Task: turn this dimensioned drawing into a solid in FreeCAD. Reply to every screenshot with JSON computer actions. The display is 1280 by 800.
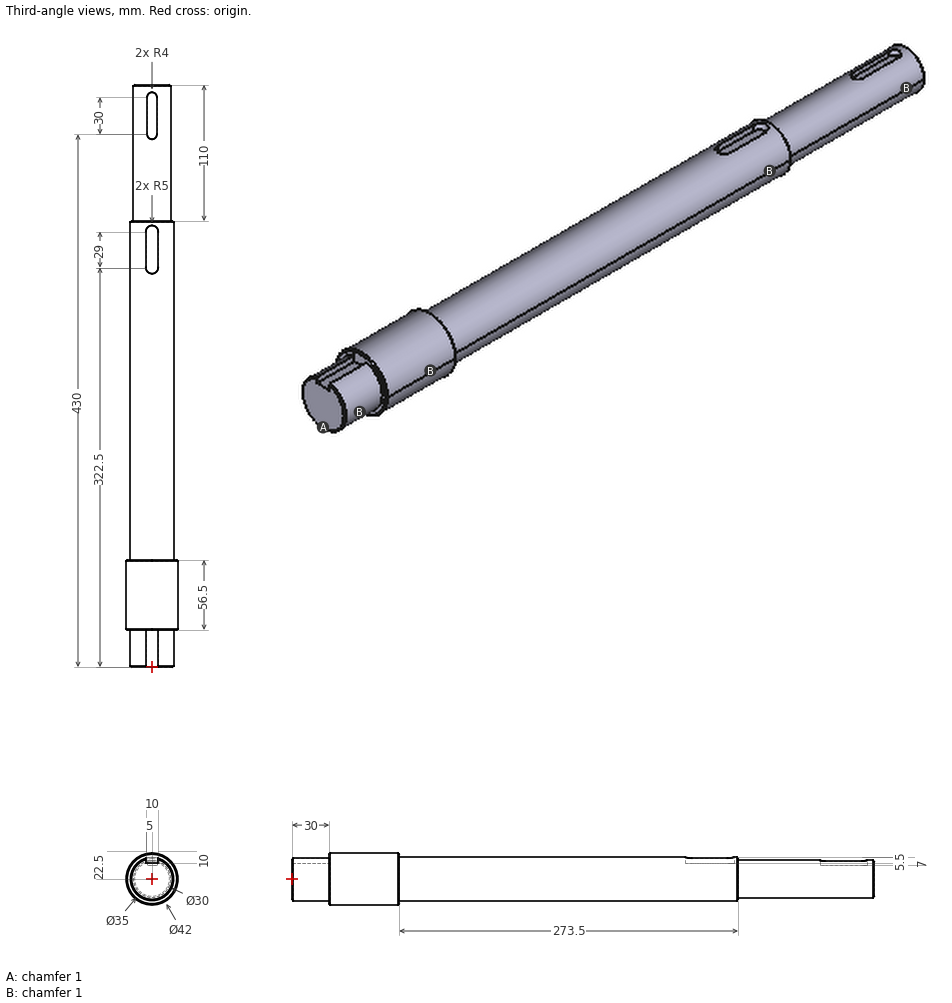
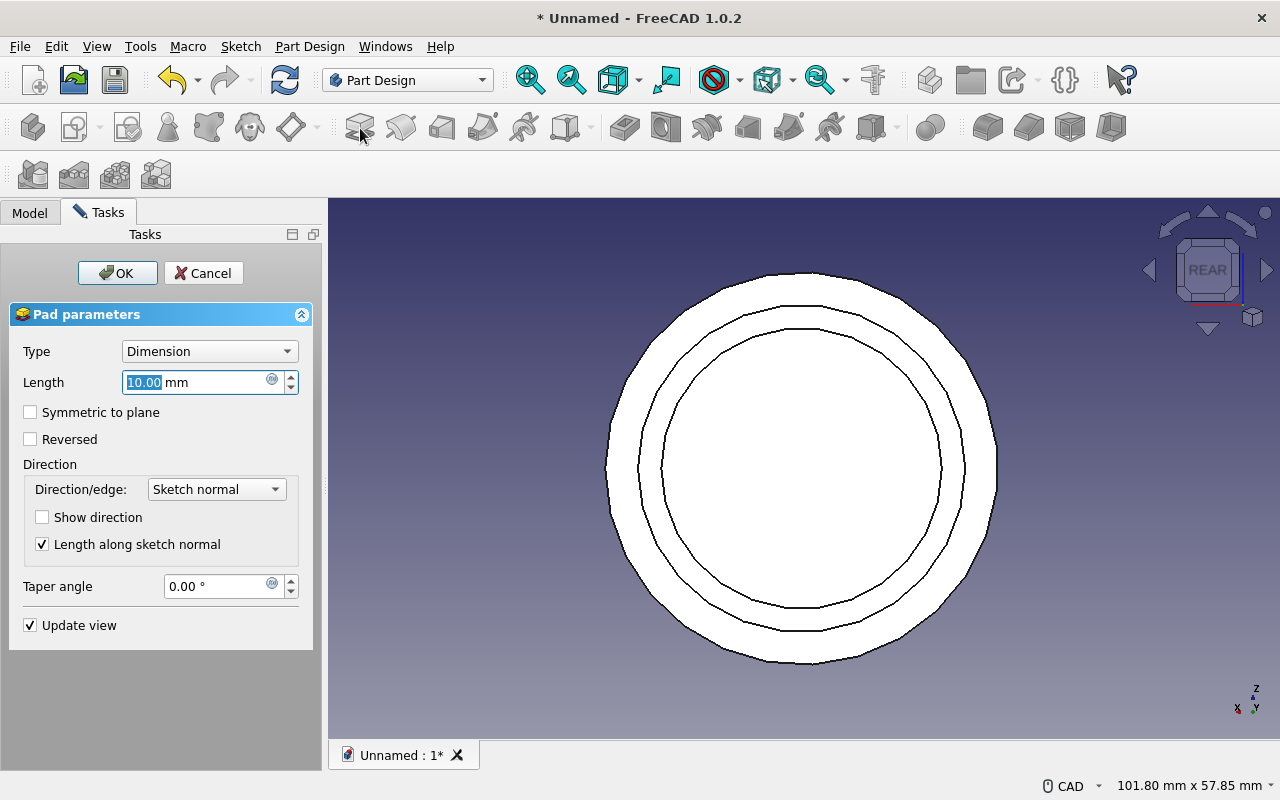
{"action": "type", "text": "110"}
{"action": "key", "text": "Tab"}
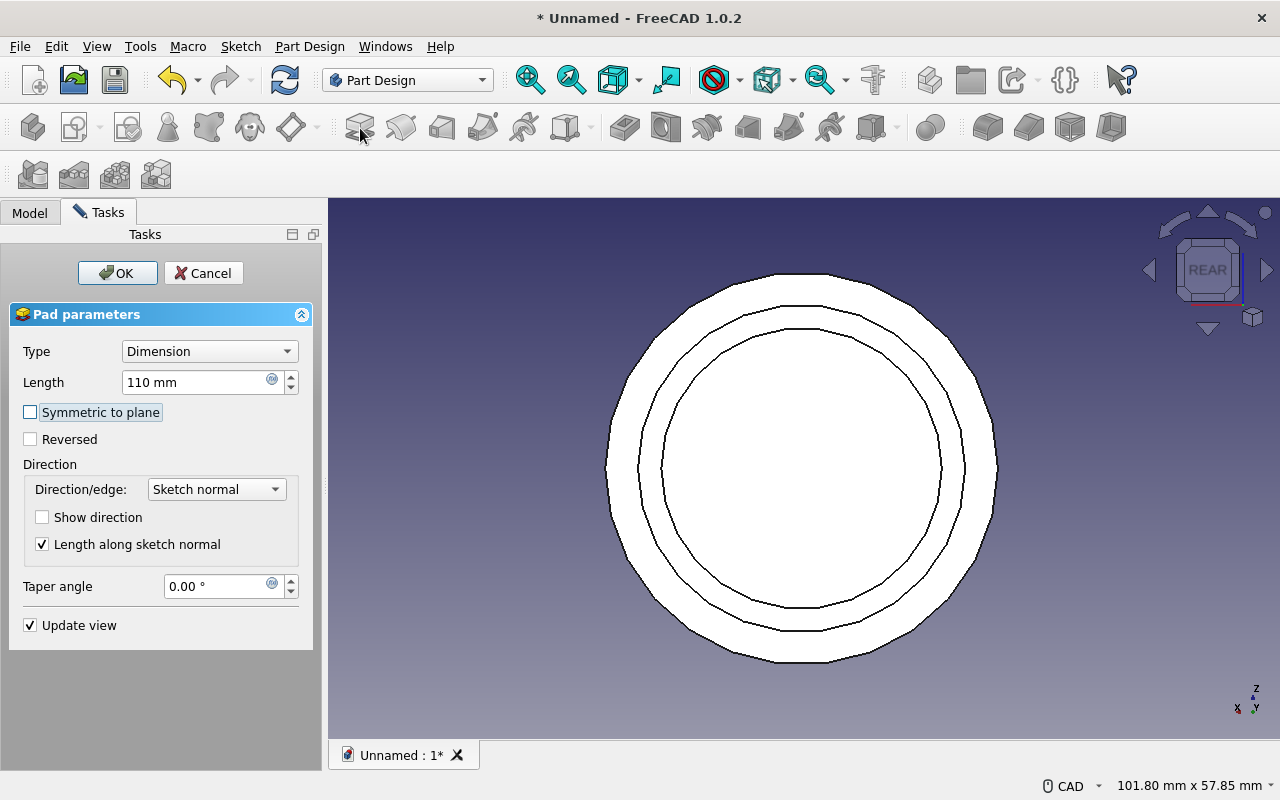
{"action": "left_click", "coordinate": [118, 273]}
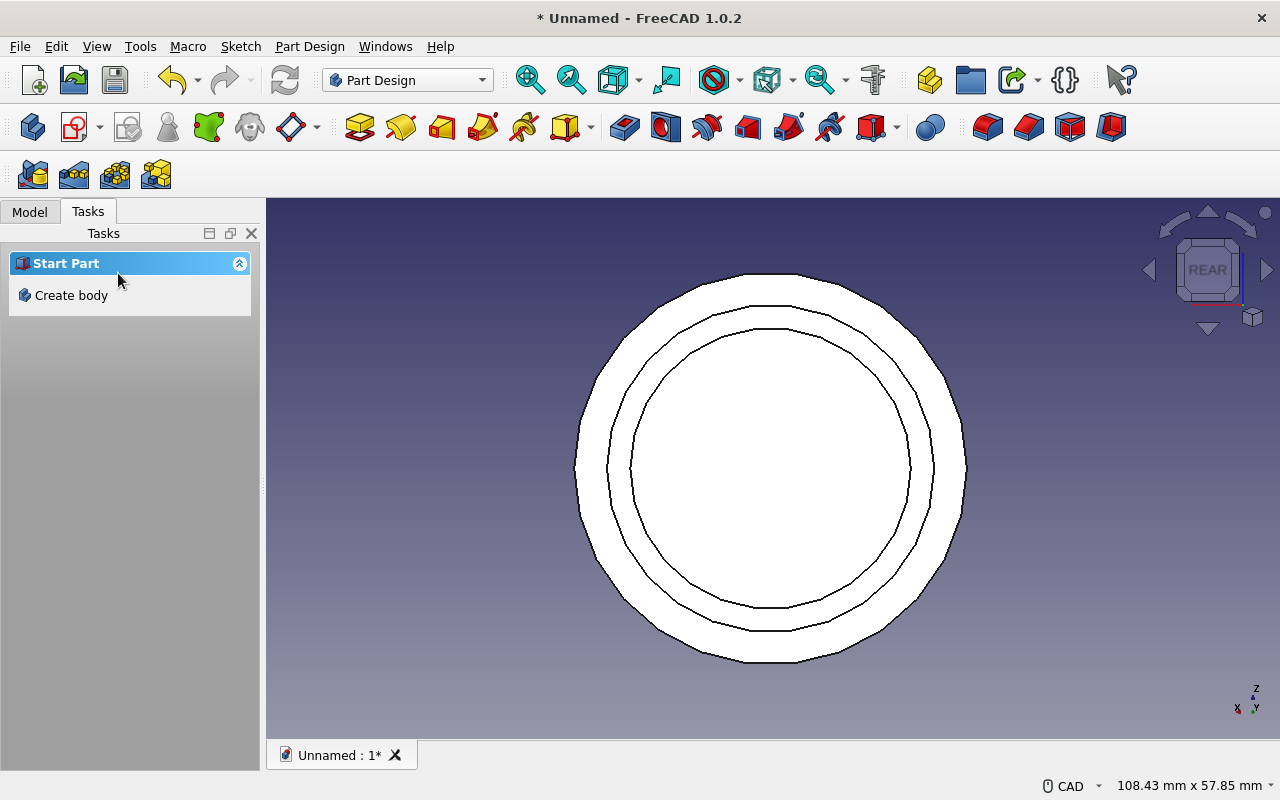
{"action": "key", "text": "0"}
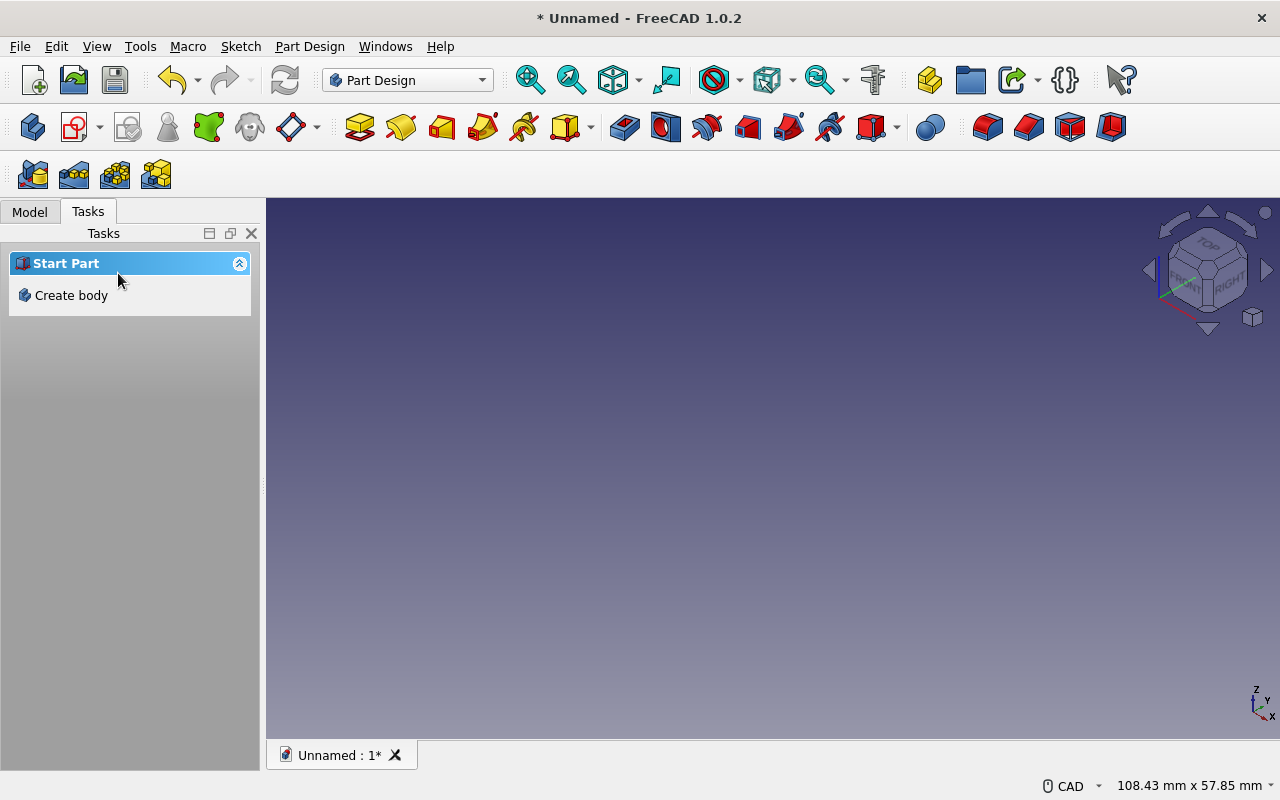
{"action": "key", "text": "v f"}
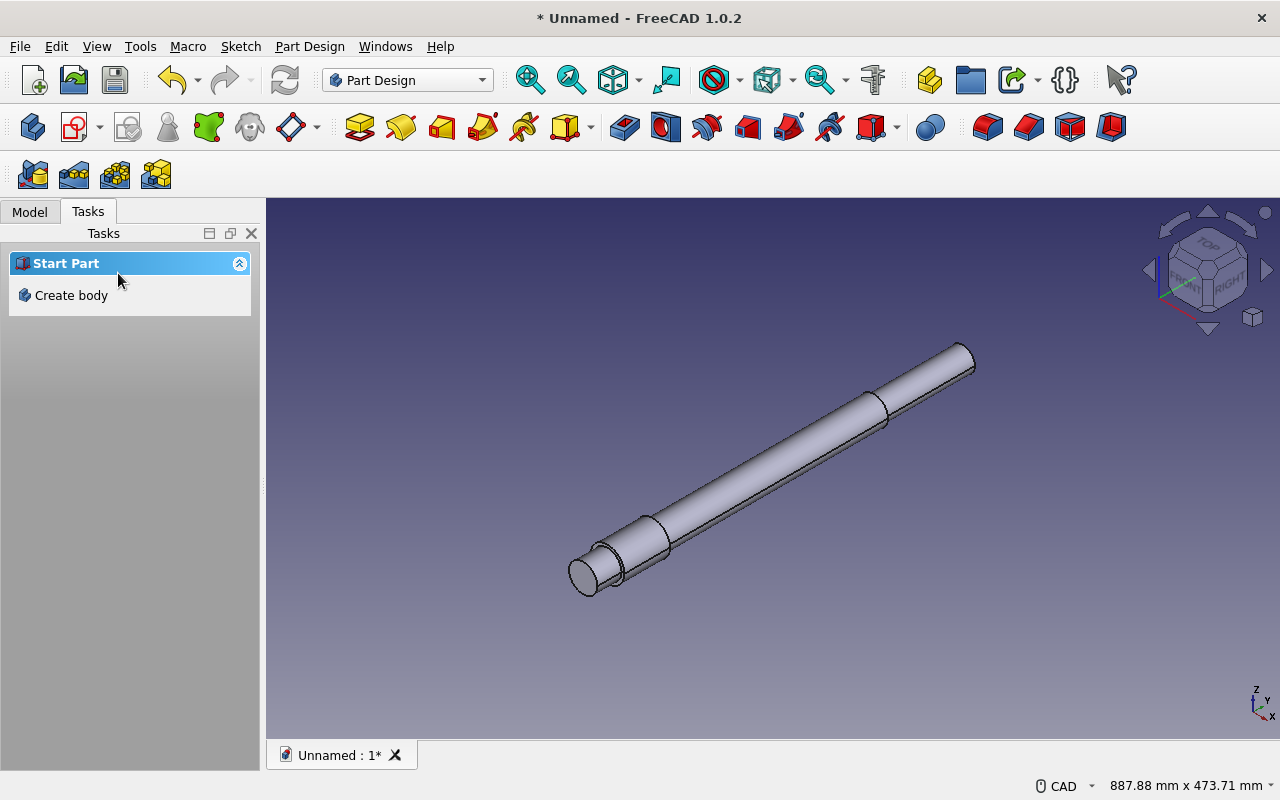
{"action": "left_click", "coordinate": [572, 561]}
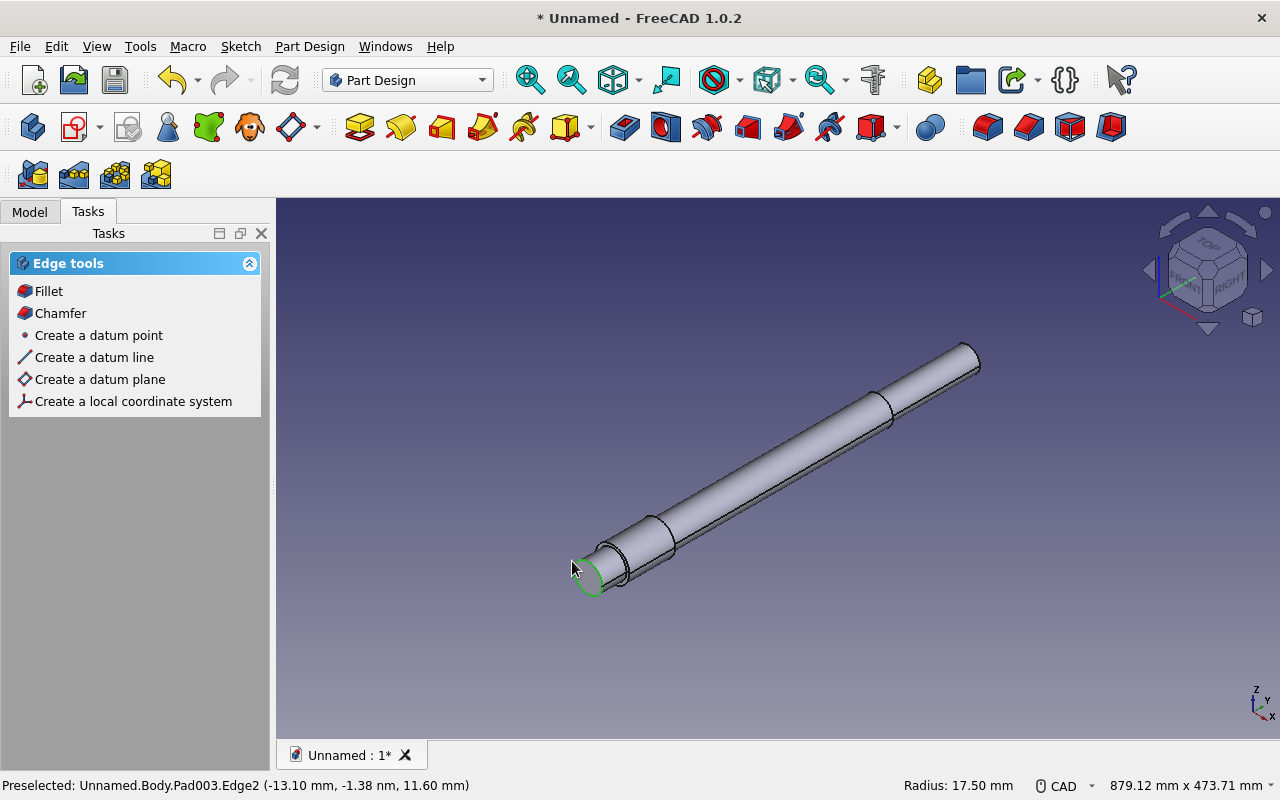
{"action": "left_click", "coordinate": [1029, 128]}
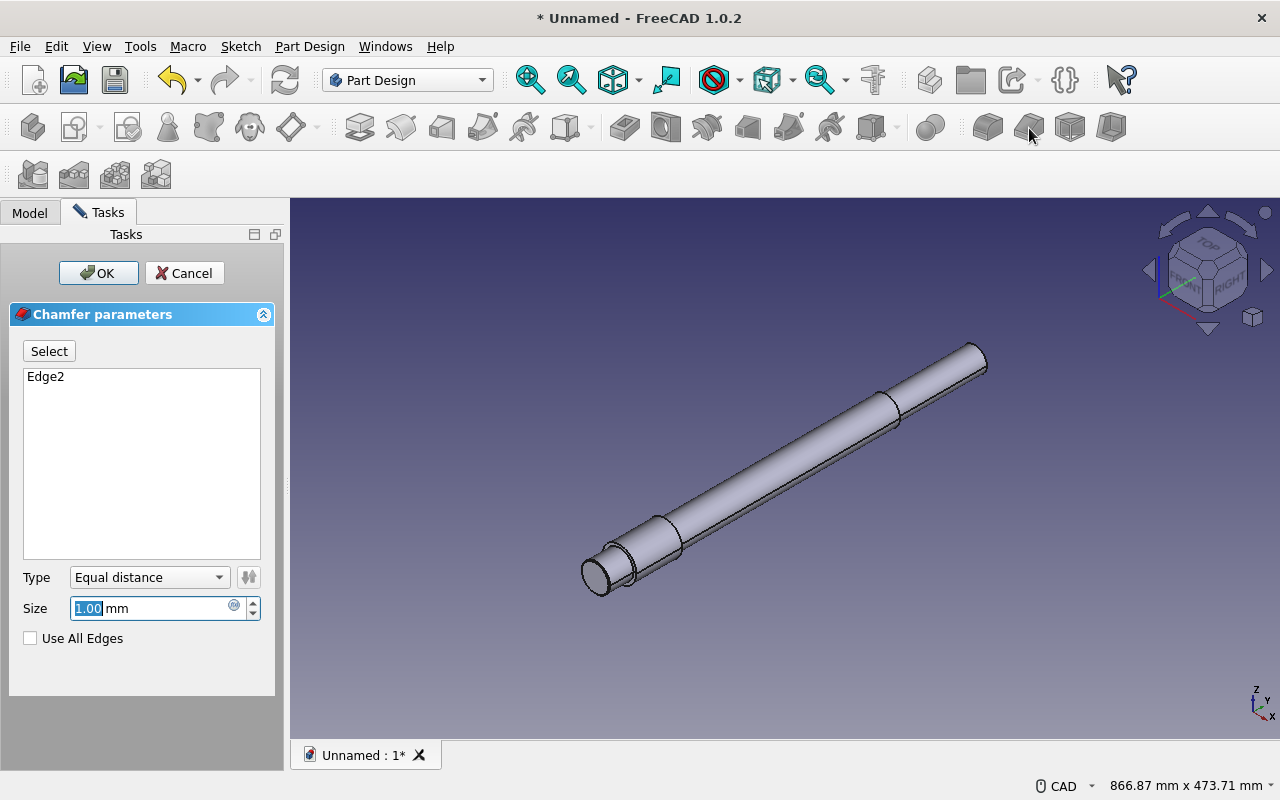
{"action": "type", "text": "1"}
{"action": "key", "text": "Tab"}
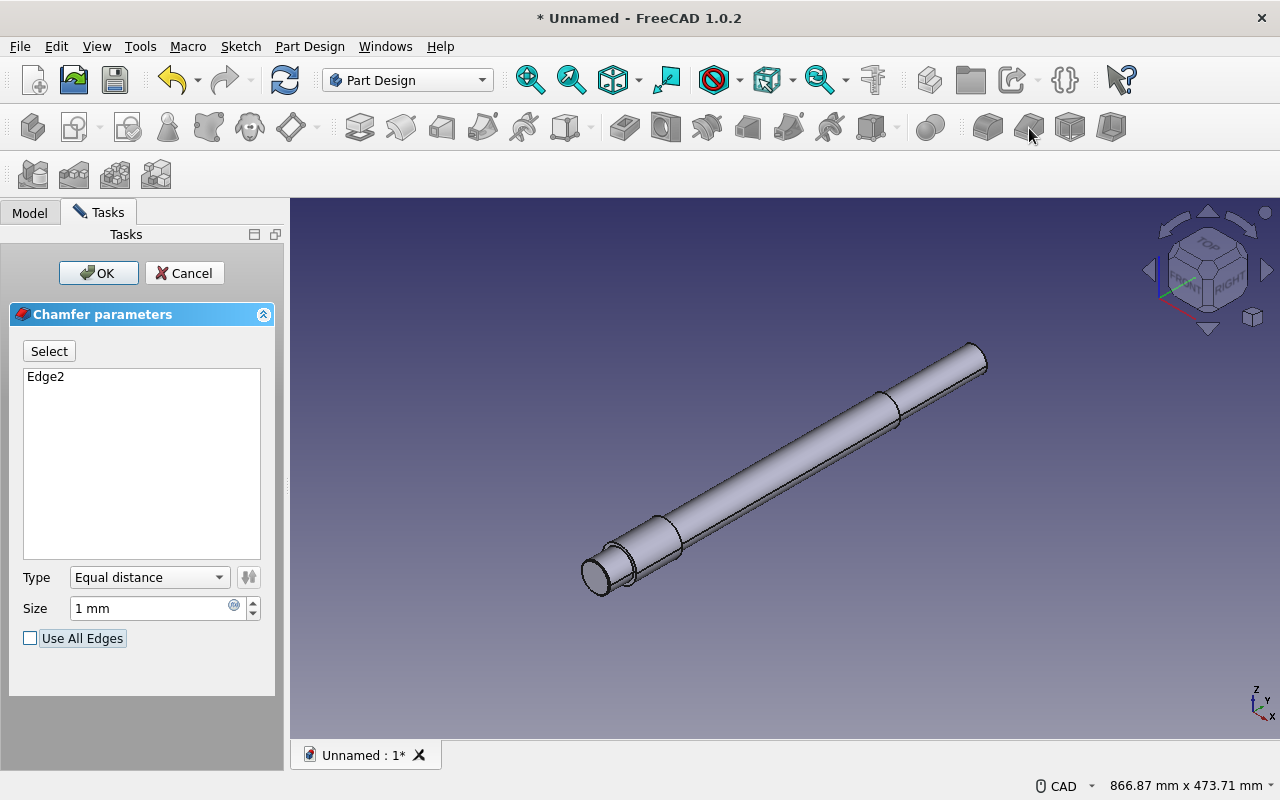
{"action": "left_click", "coordinate": [99, 273]}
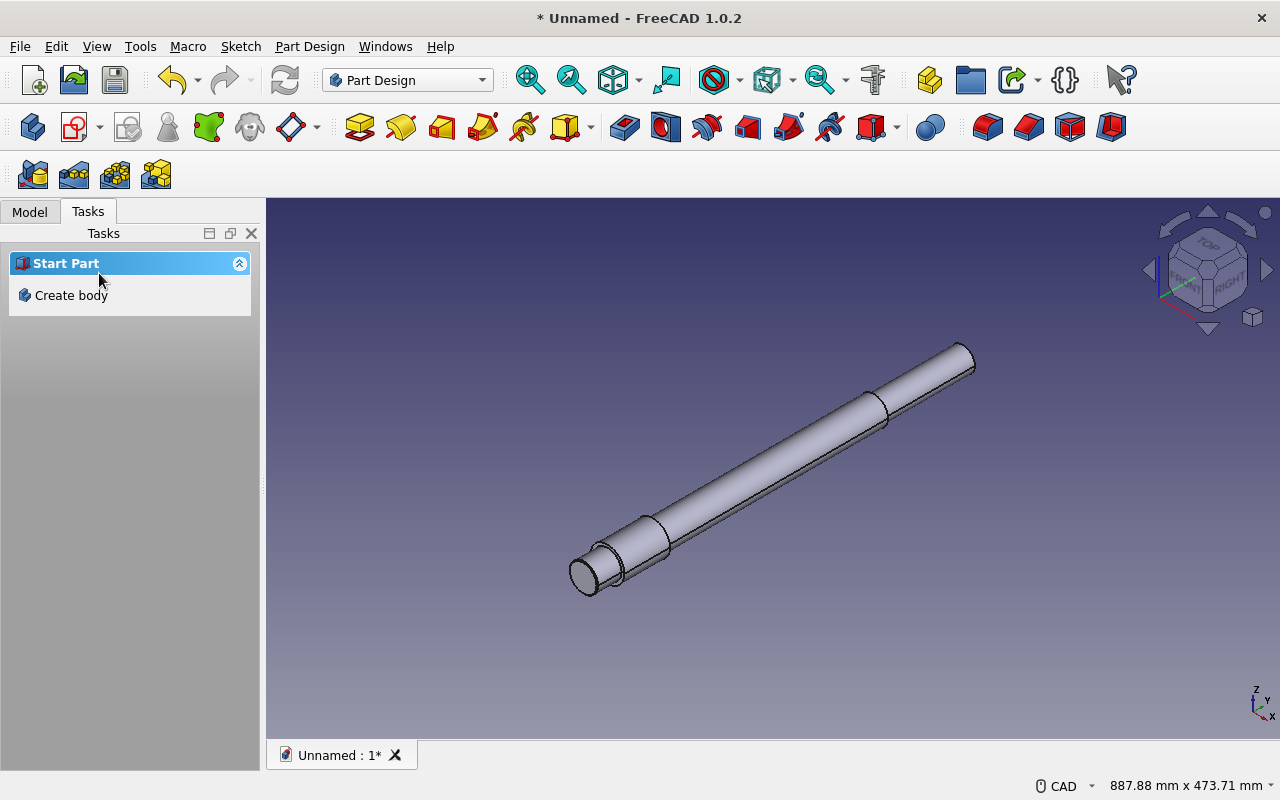
{"action": "left_click", "coordinate": [870, 391]}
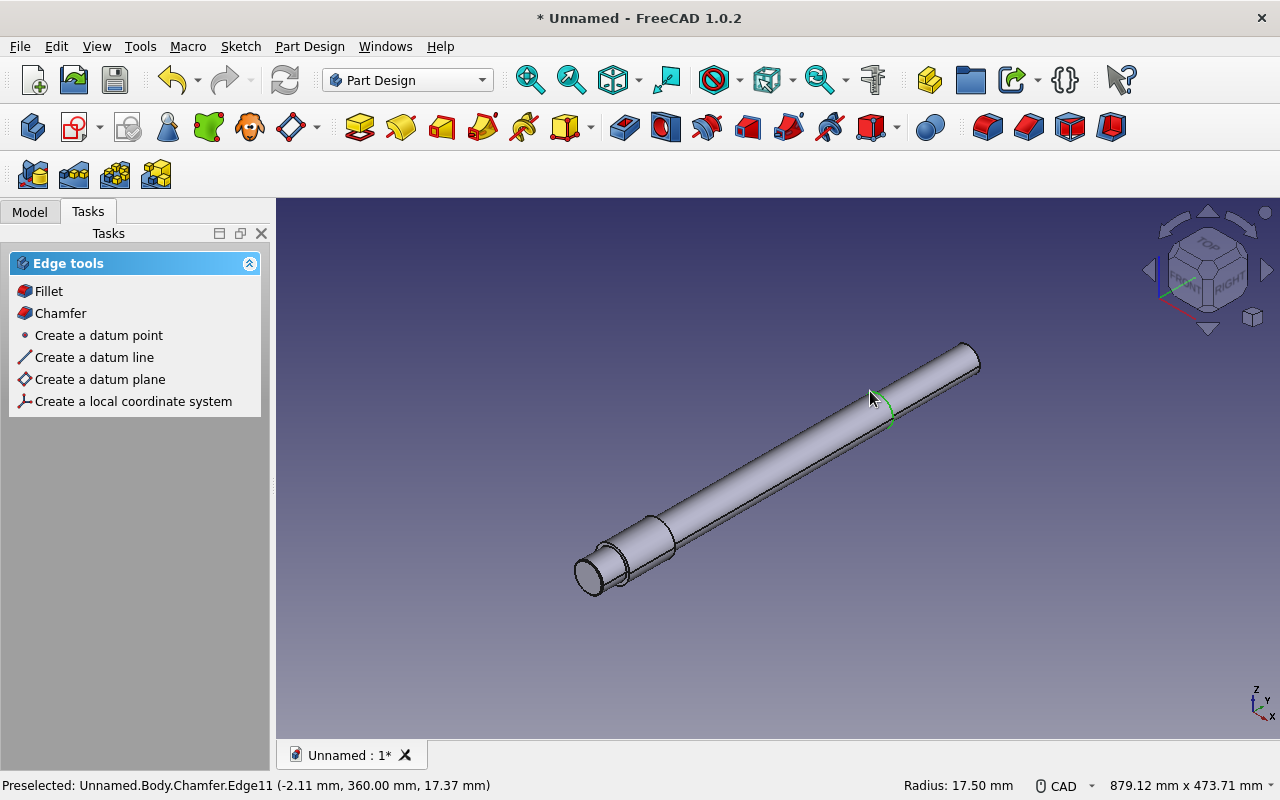
{"action": "left_click", "coordinate": [964, 342], "text": "ctrl"}